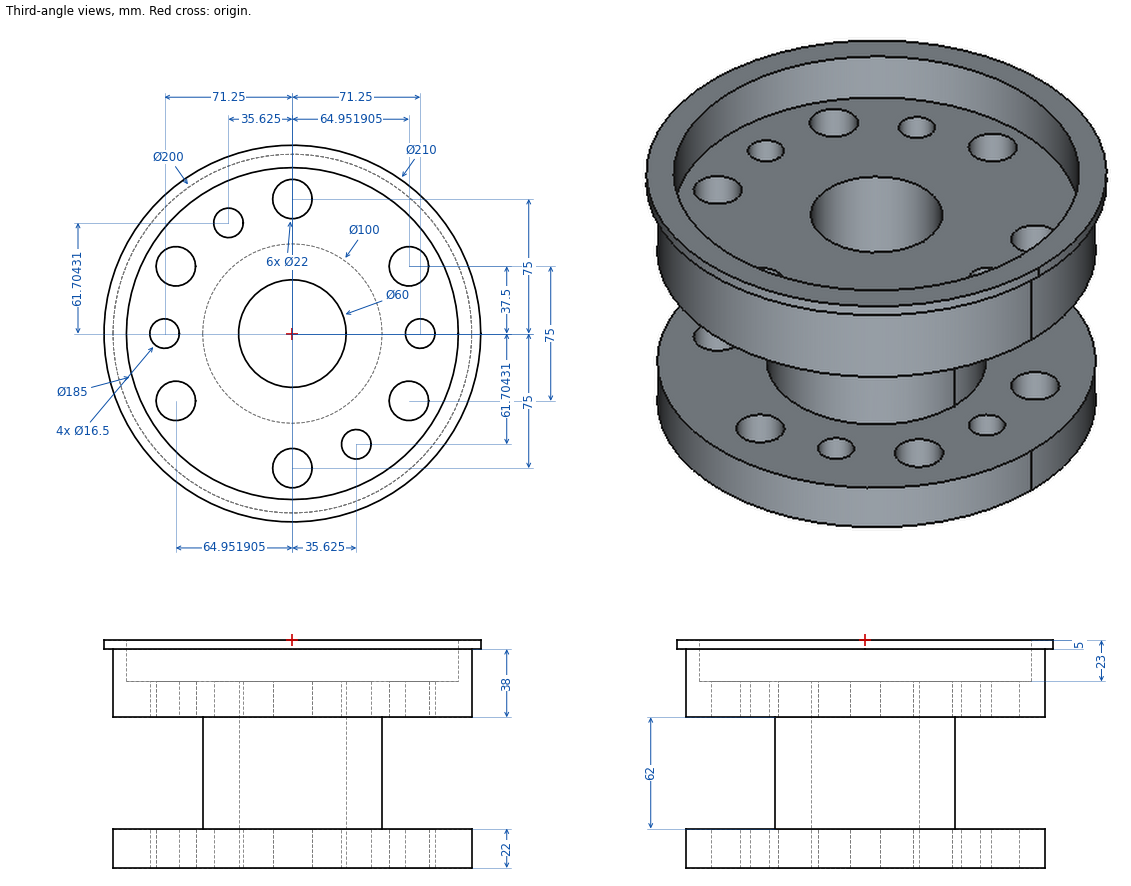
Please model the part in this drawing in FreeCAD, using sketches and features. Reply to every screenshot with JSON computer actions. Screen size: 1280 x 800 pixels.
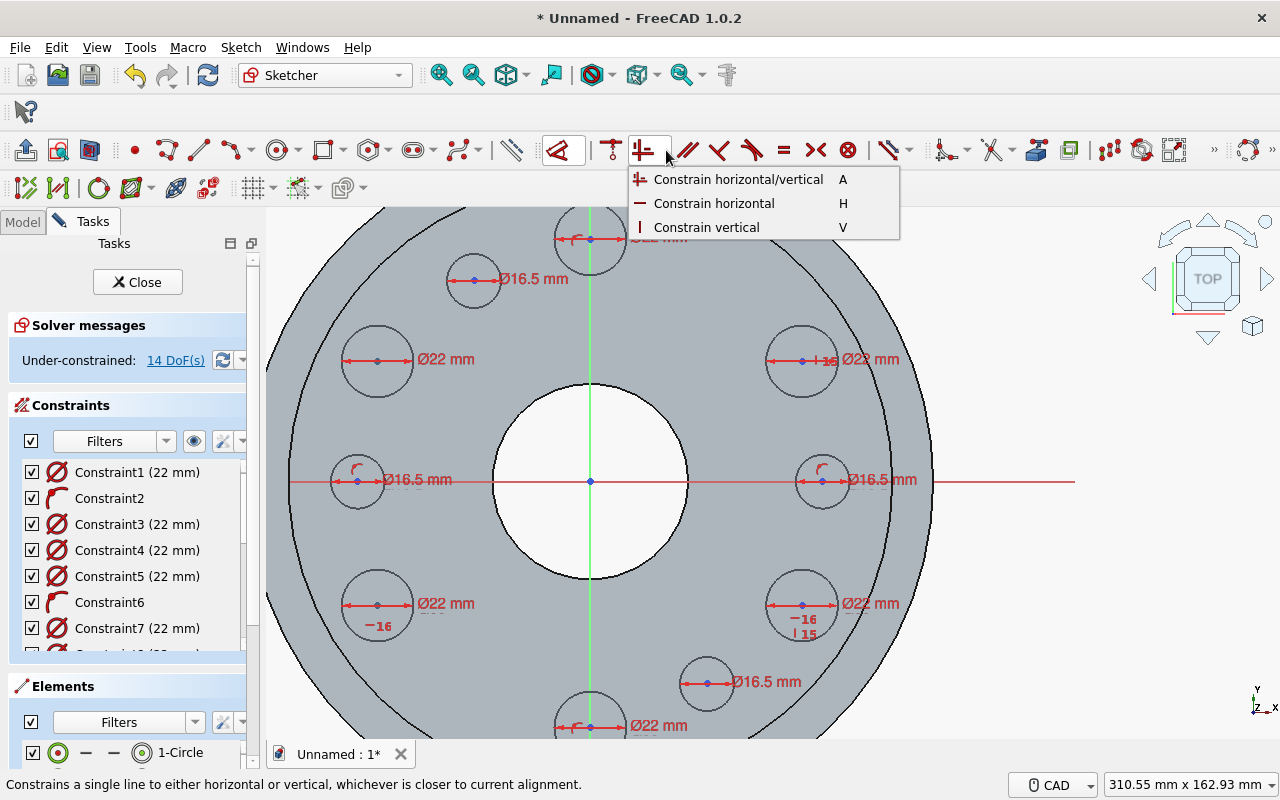
{"action": "left_click", "coordinate": [764, 227]}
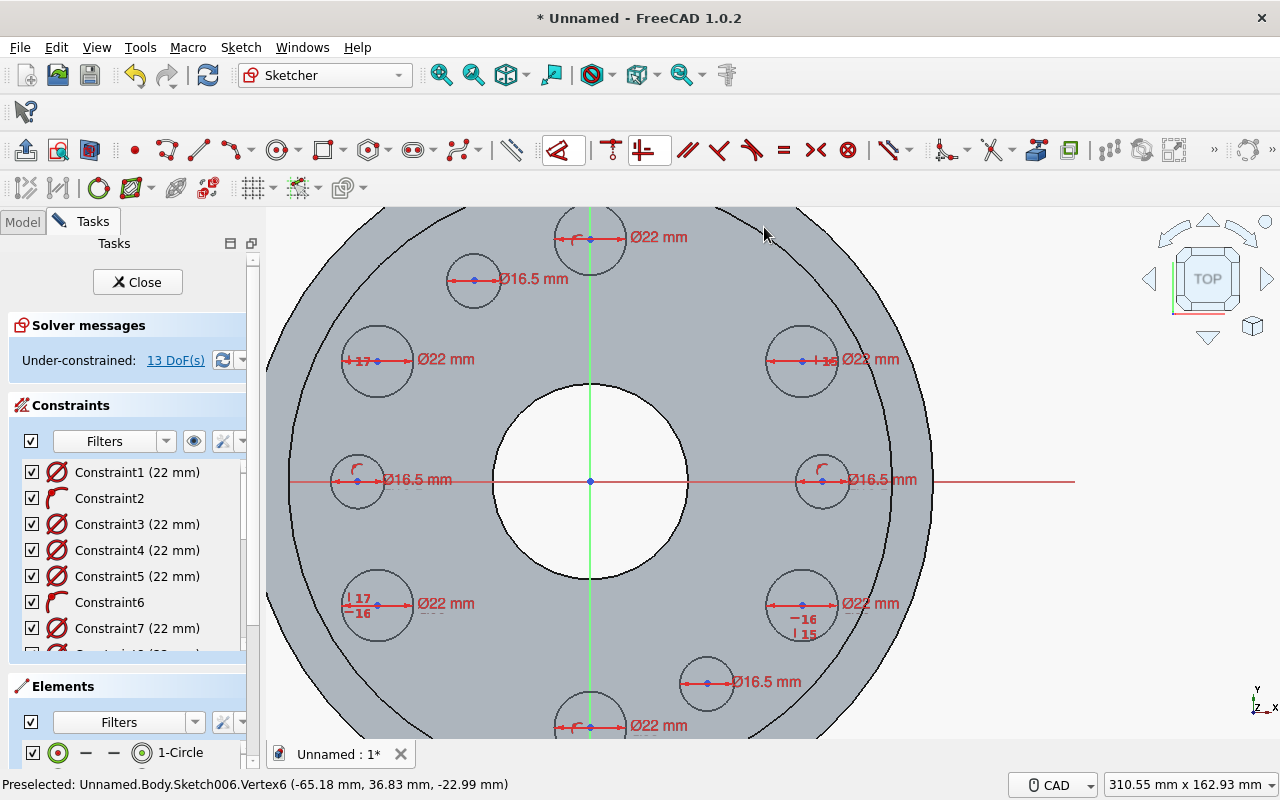
{"action": "left_click", "coordinate": [802, 361]}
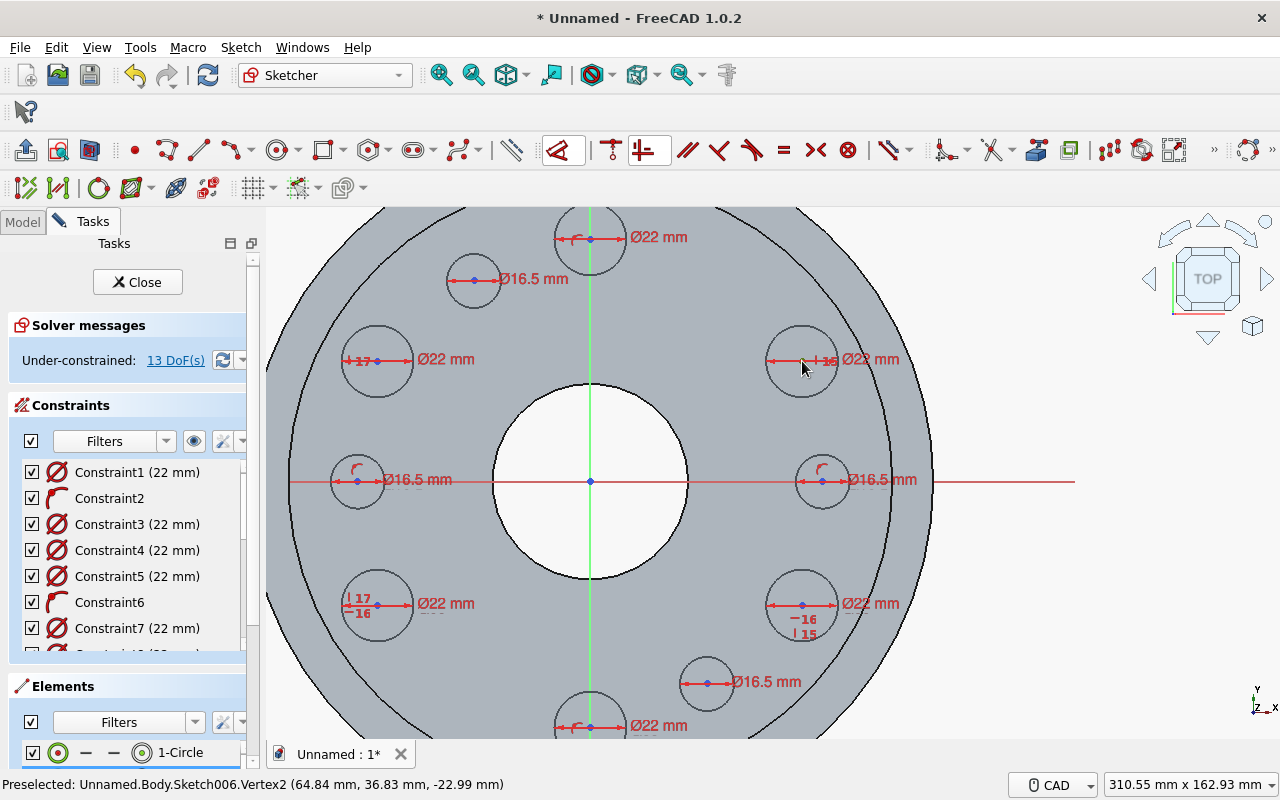
{"action": "left_click", "coordinate": [378, 361]}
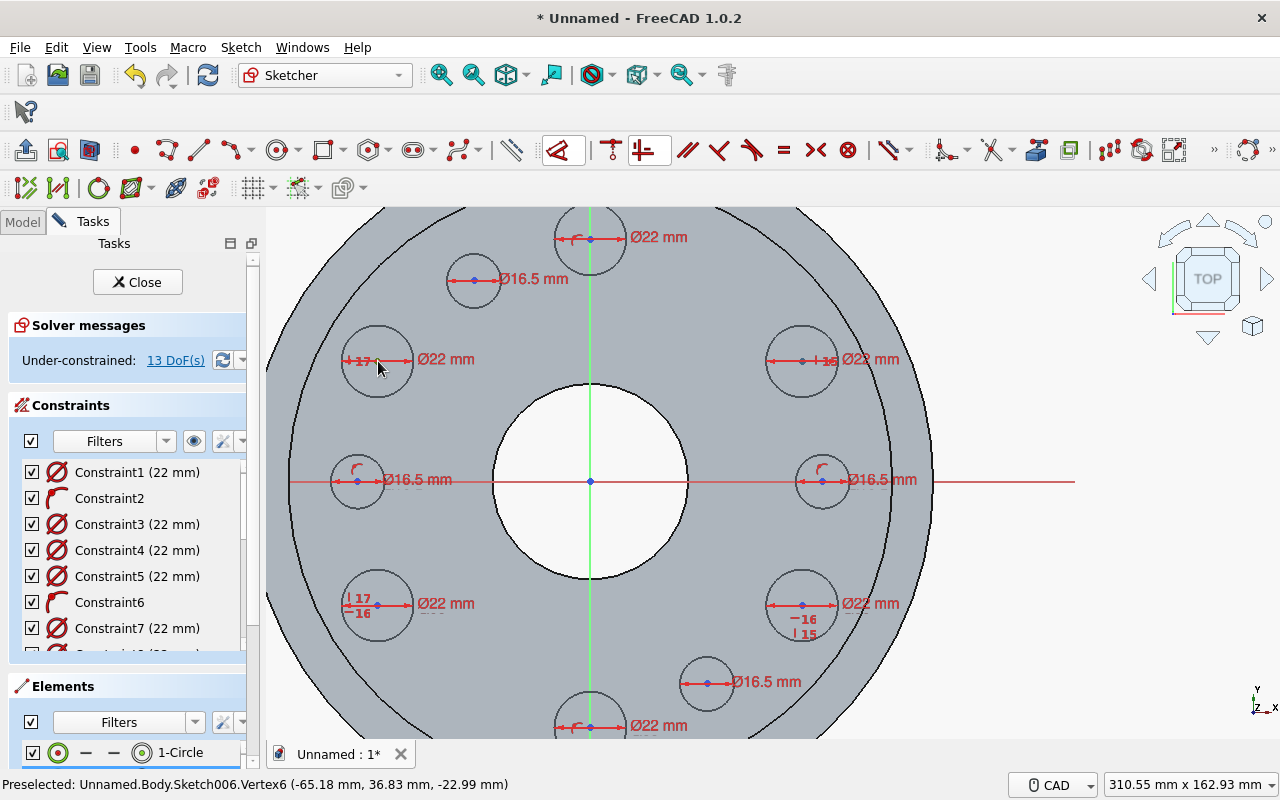
{"action": "left_click", "coordinate": [666, 150]}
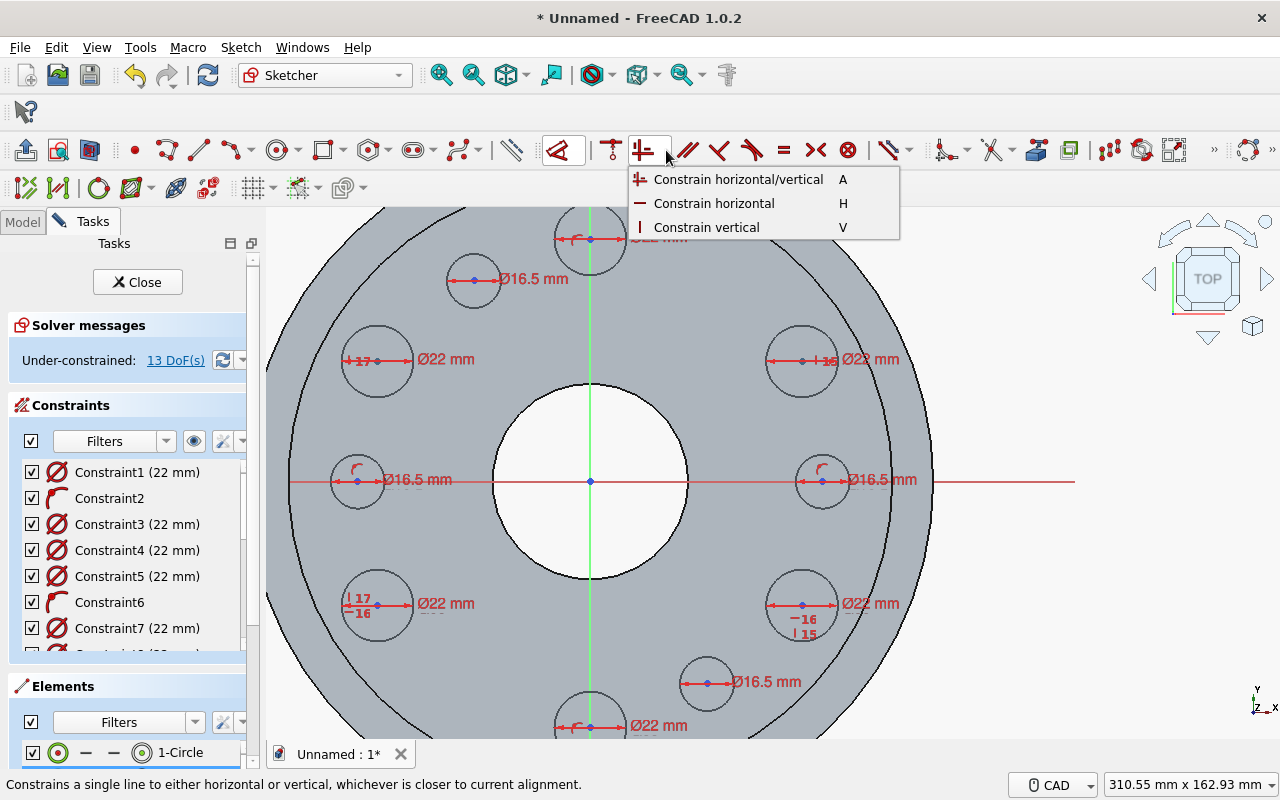
{"action": "left_click", "coordinate": [764, 203]}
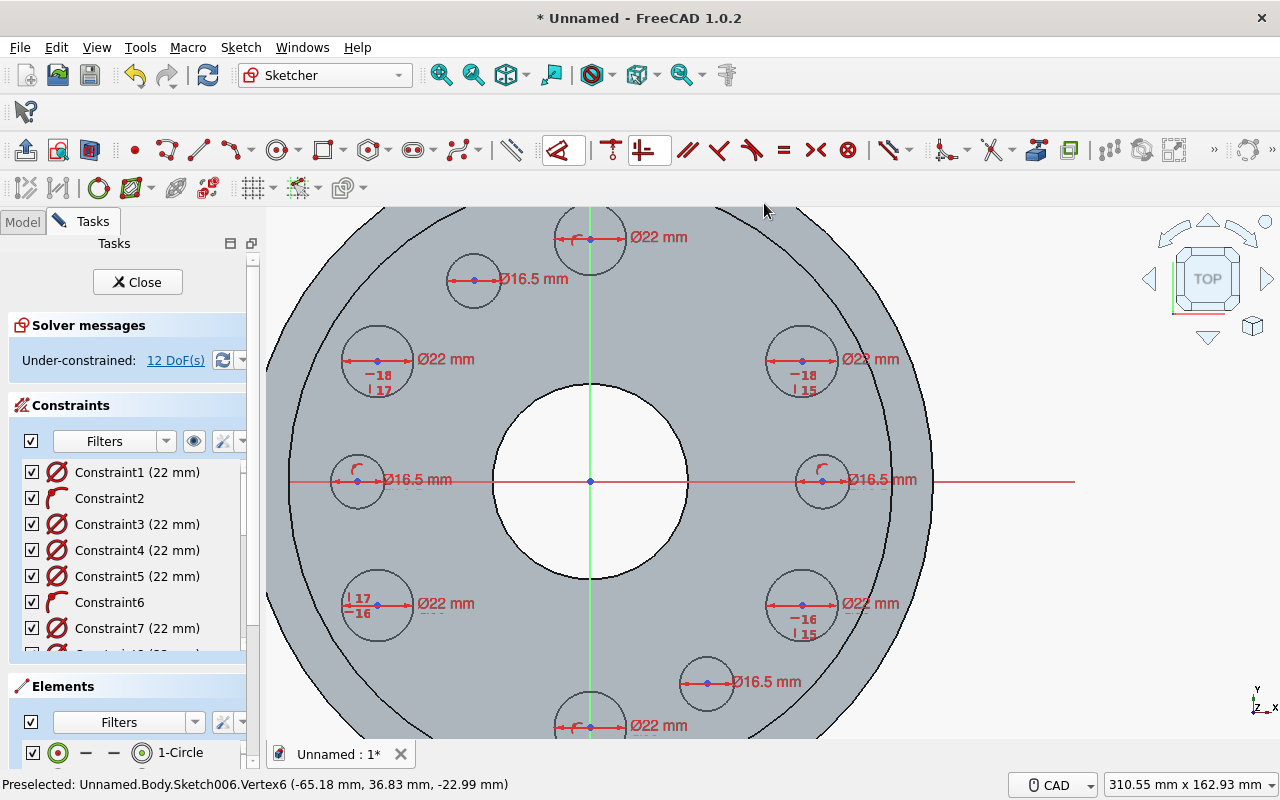
{"action": "left_click", "coordinate": [558, 150]}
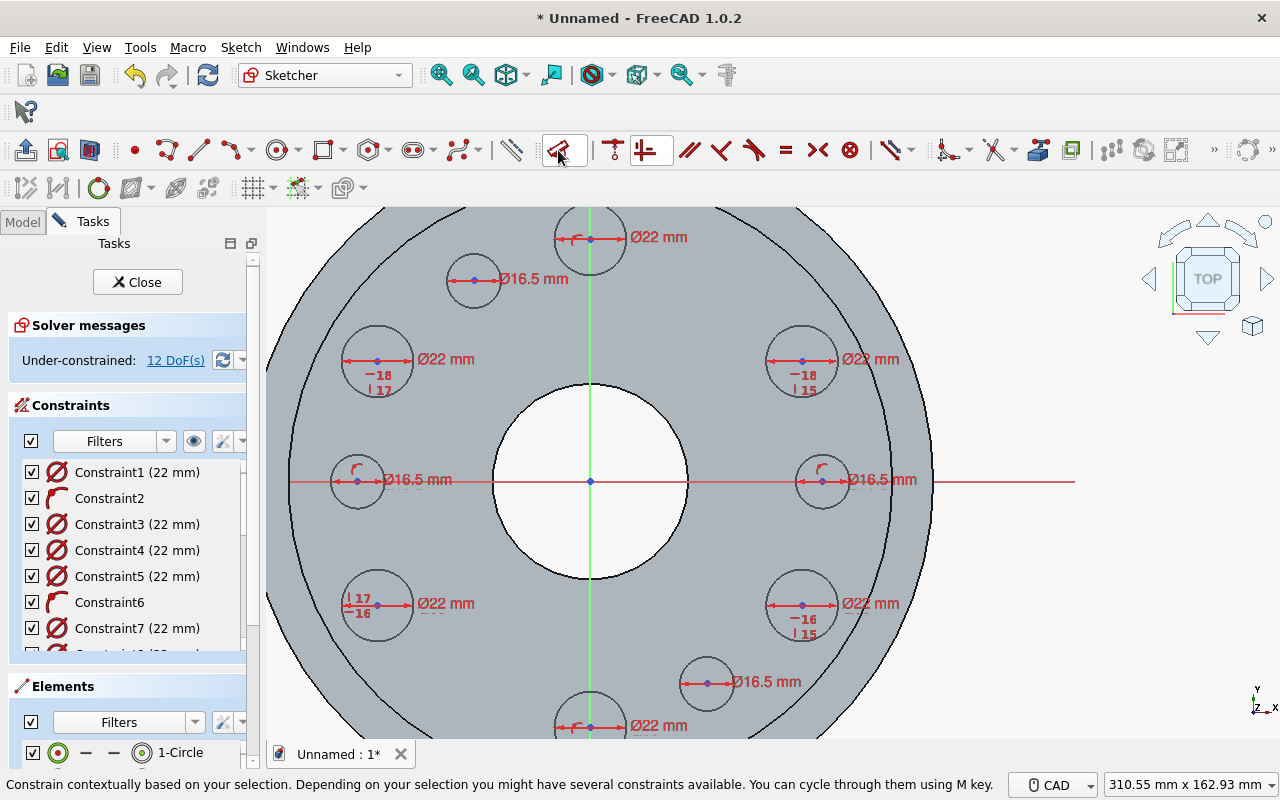
{"action": "left_click", "coordinate": [590, 239]}
{"action": "left_click", "coordinate": [624, 360]}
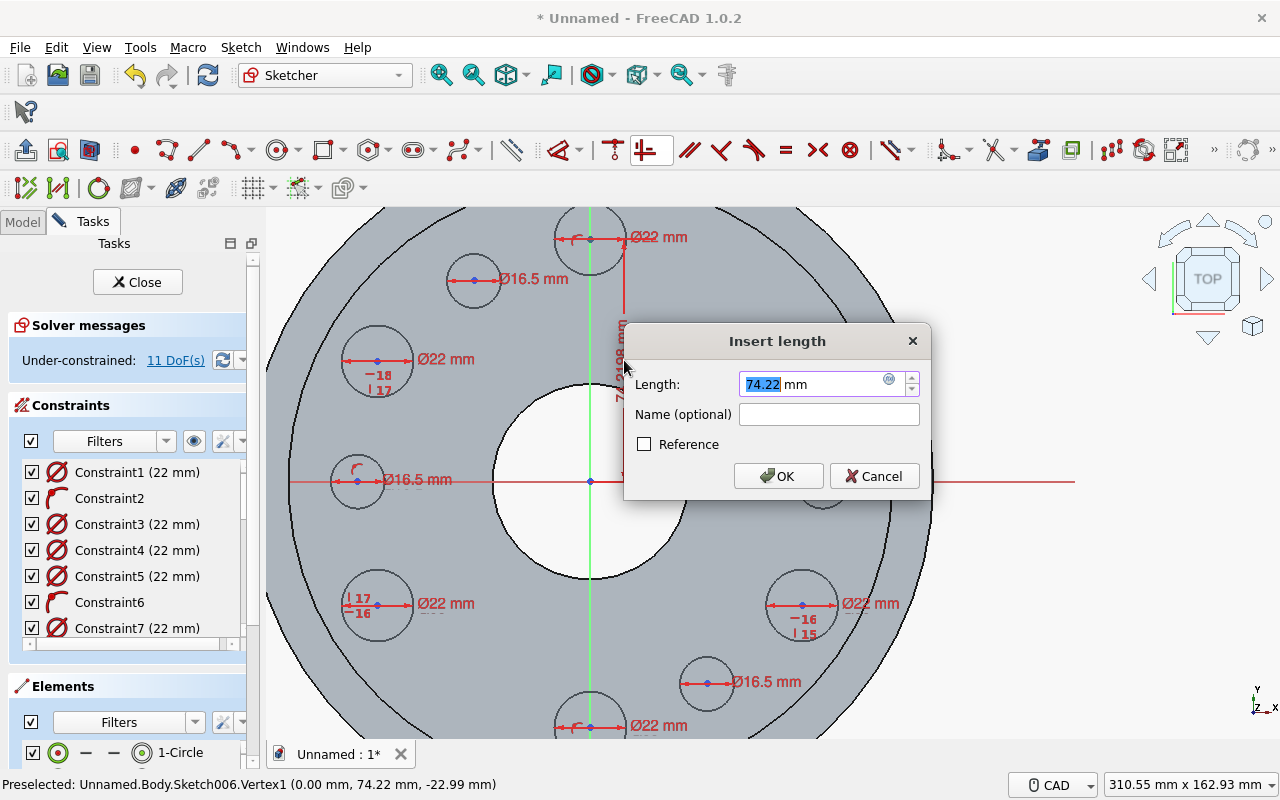
{"action": "type", "text": "75"}
{"action": "key", "text": "Return"}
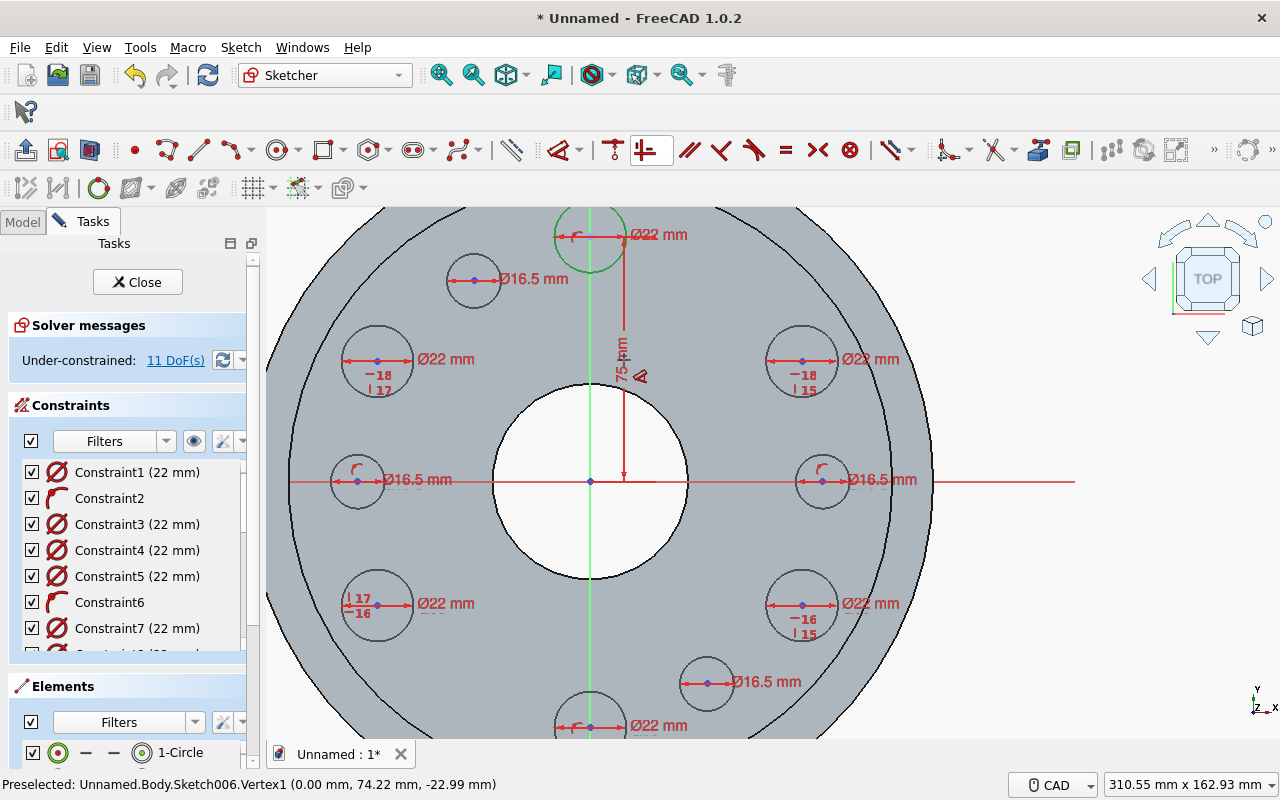
{"action": "scroll", "coordinate": [843, 462], "scroll_direction": "down", "scroll_amount": 3}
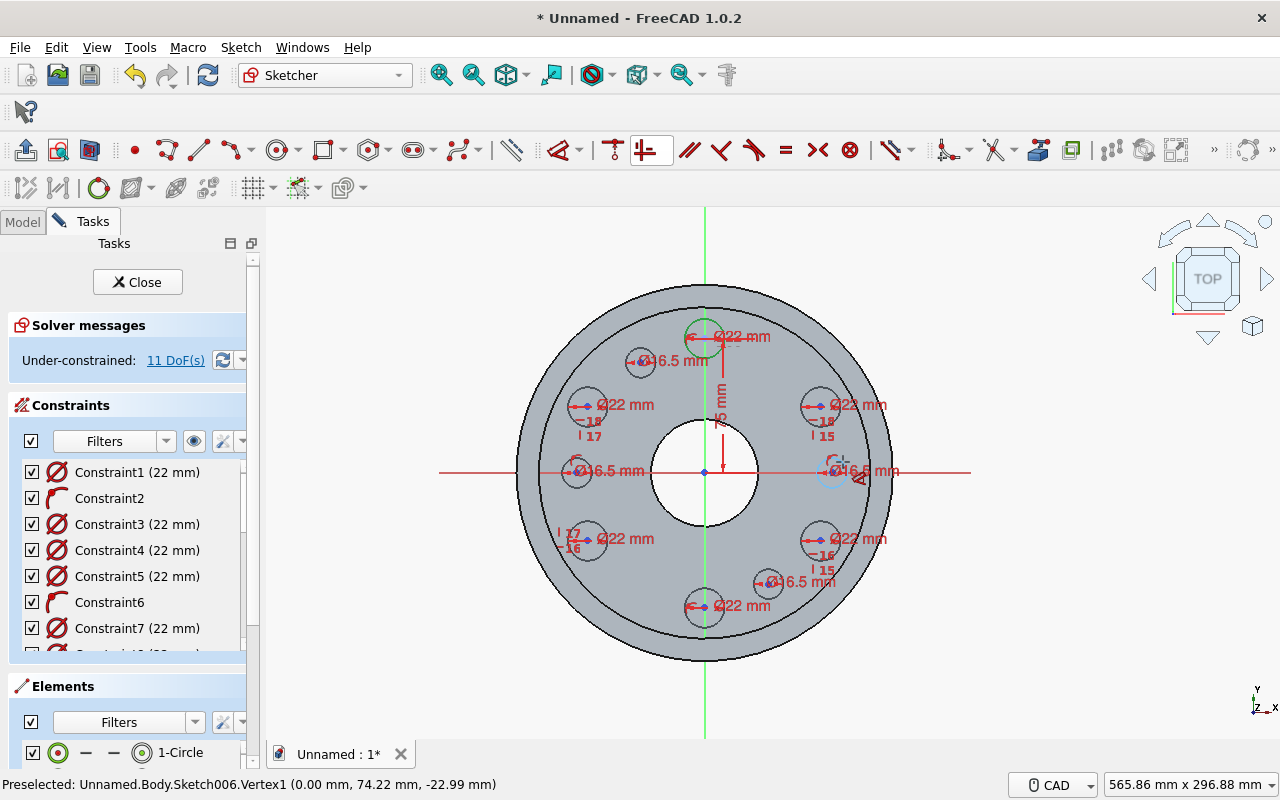
{"action": "left_click", "coordinate": [705, 608]}
{"action": "left_click", "coordinate": [739, 540]}